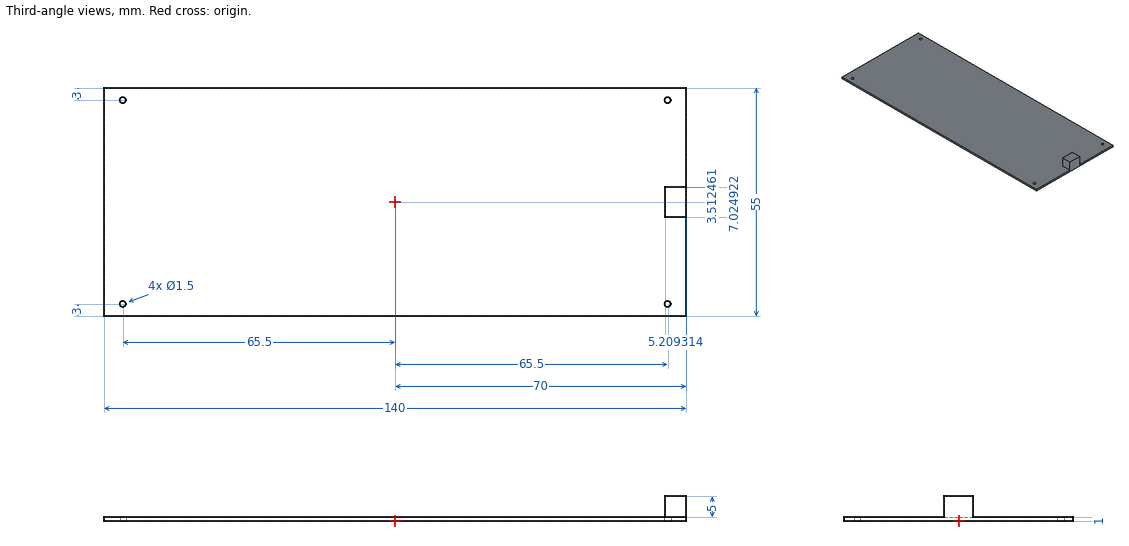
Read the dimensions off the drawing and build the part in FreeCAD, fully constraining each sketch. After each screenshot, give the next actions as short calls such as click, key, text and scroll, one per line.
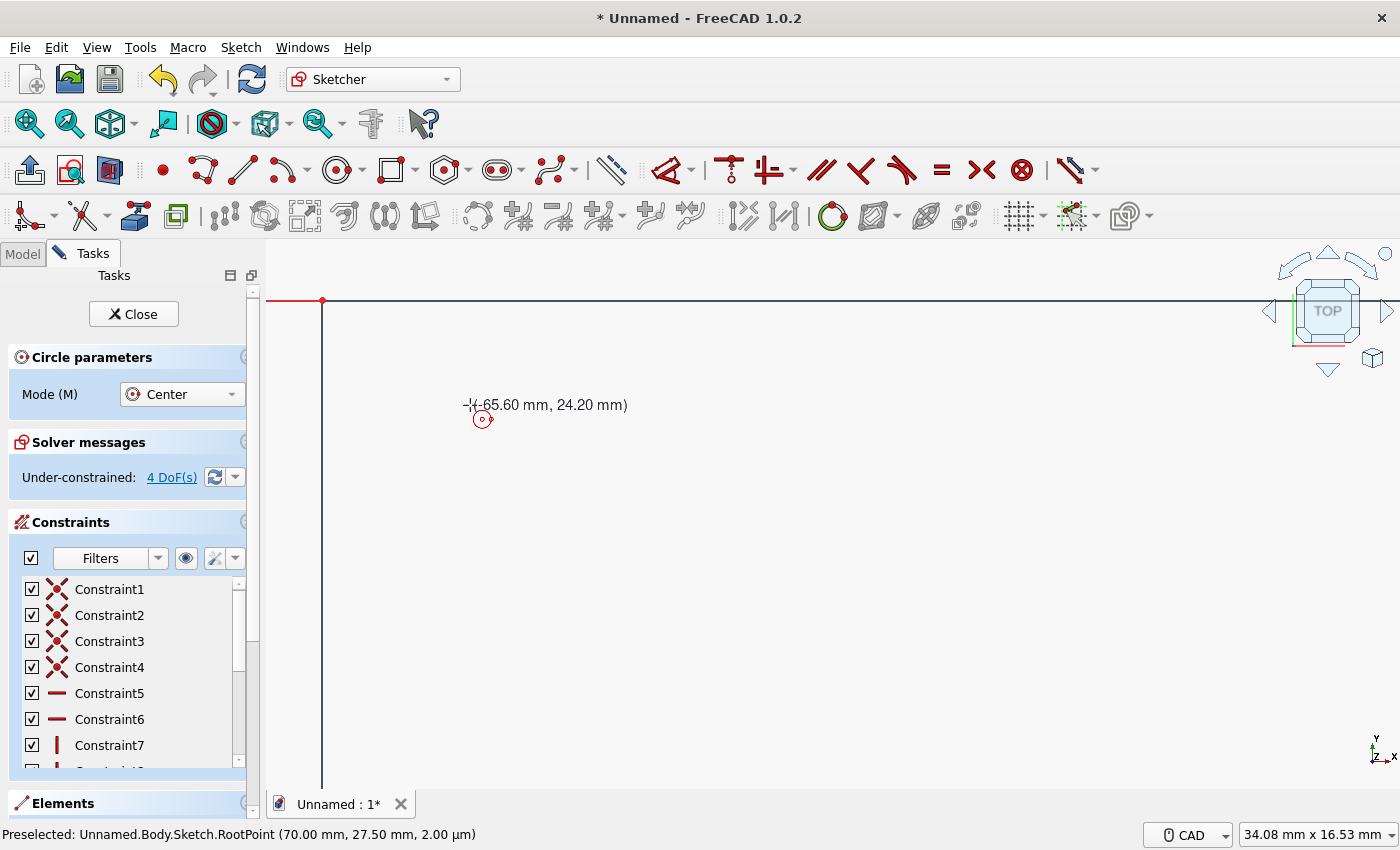
scroll(469, 404, down, 10)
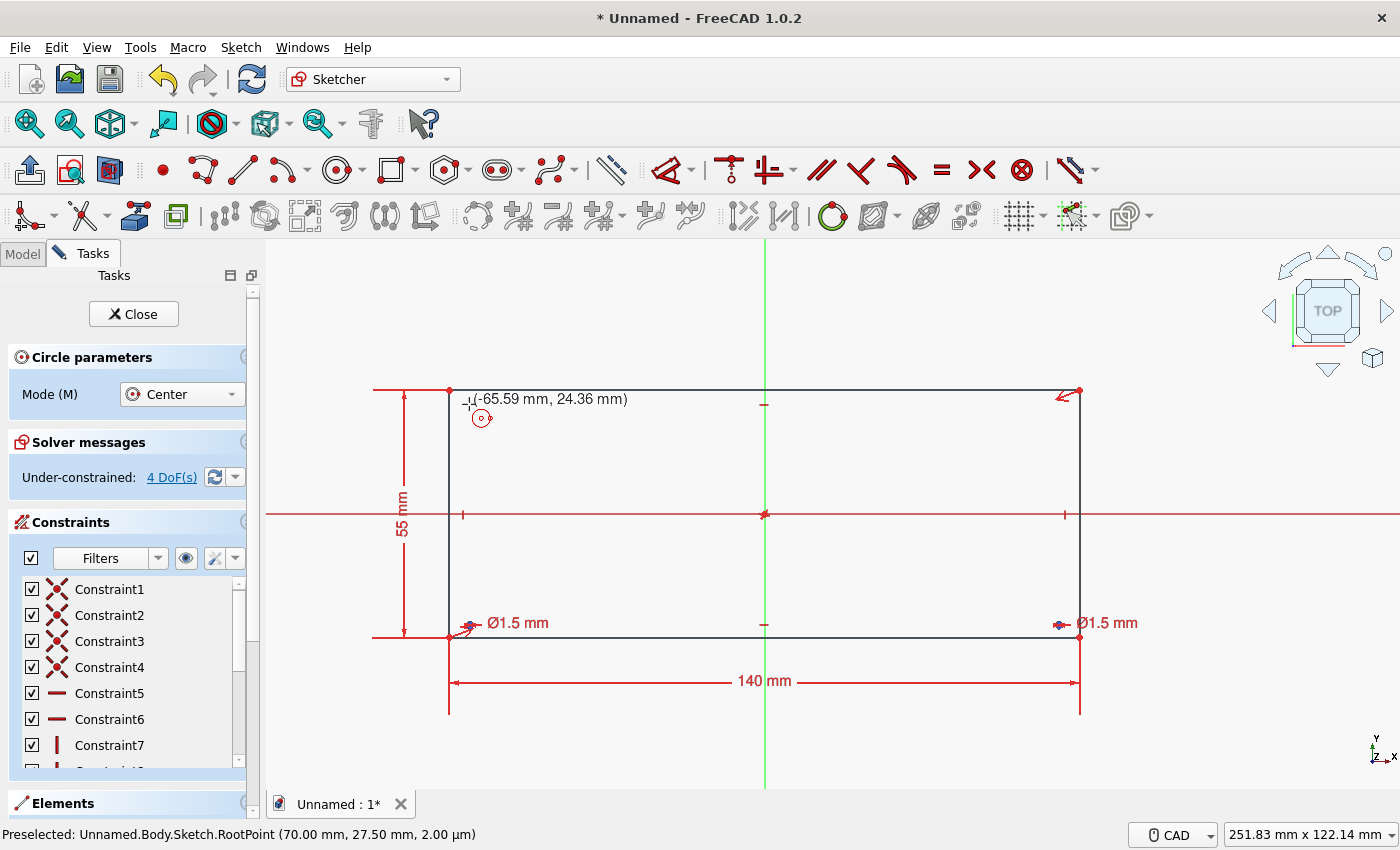
click(470, 404)
move(472, 406)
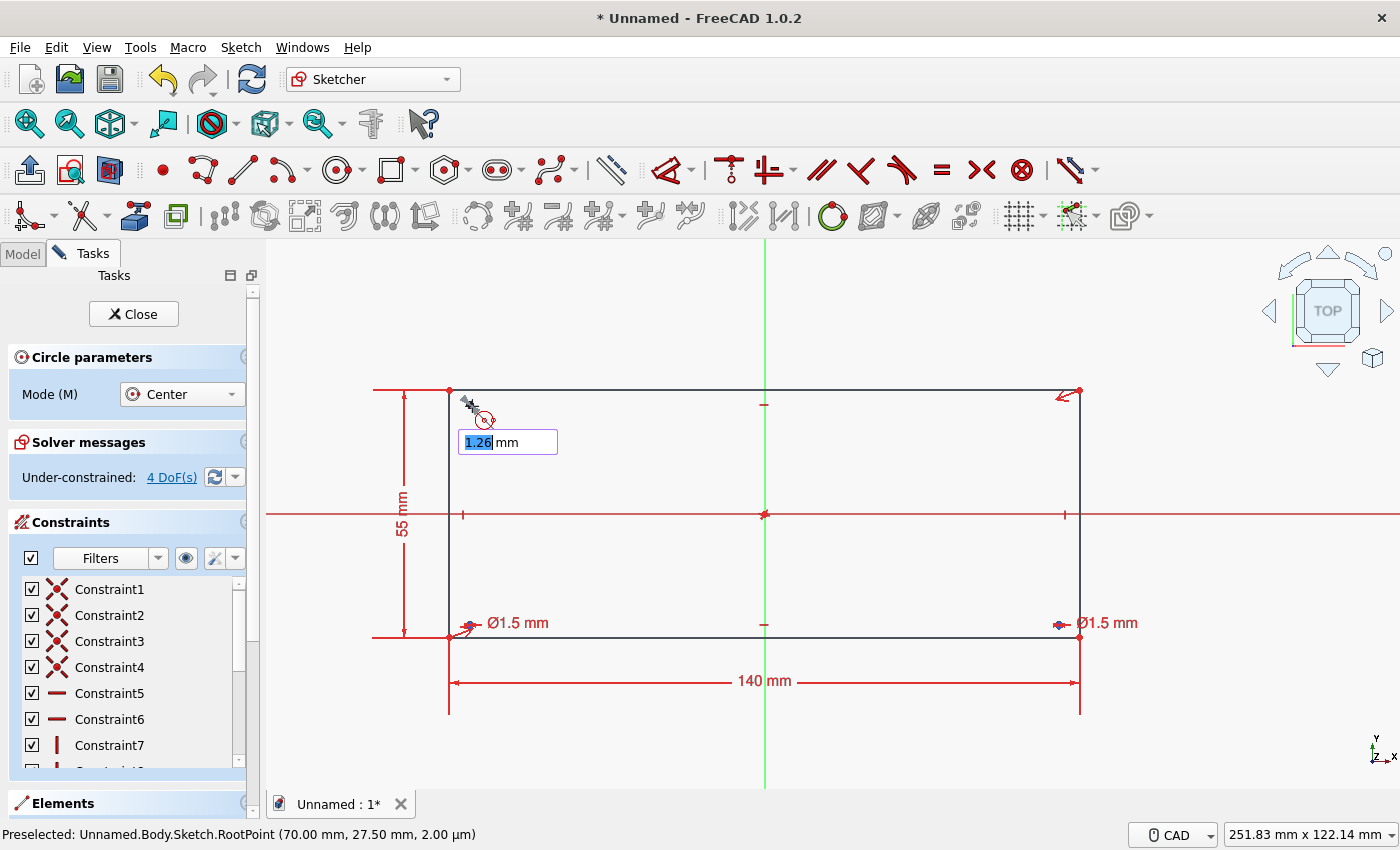
text(1.5)
key(Return)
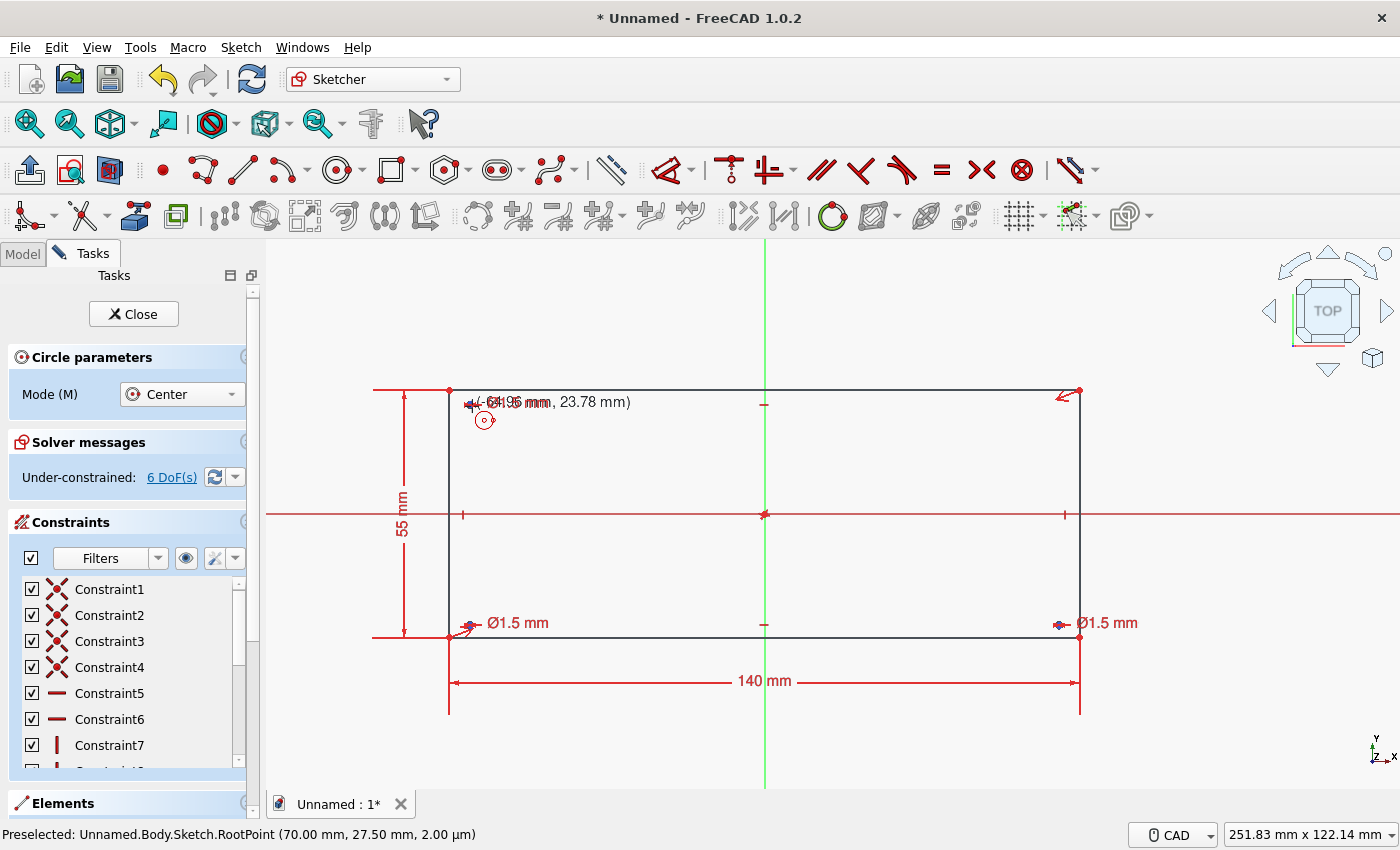
scroll(1059, 404, up, 10)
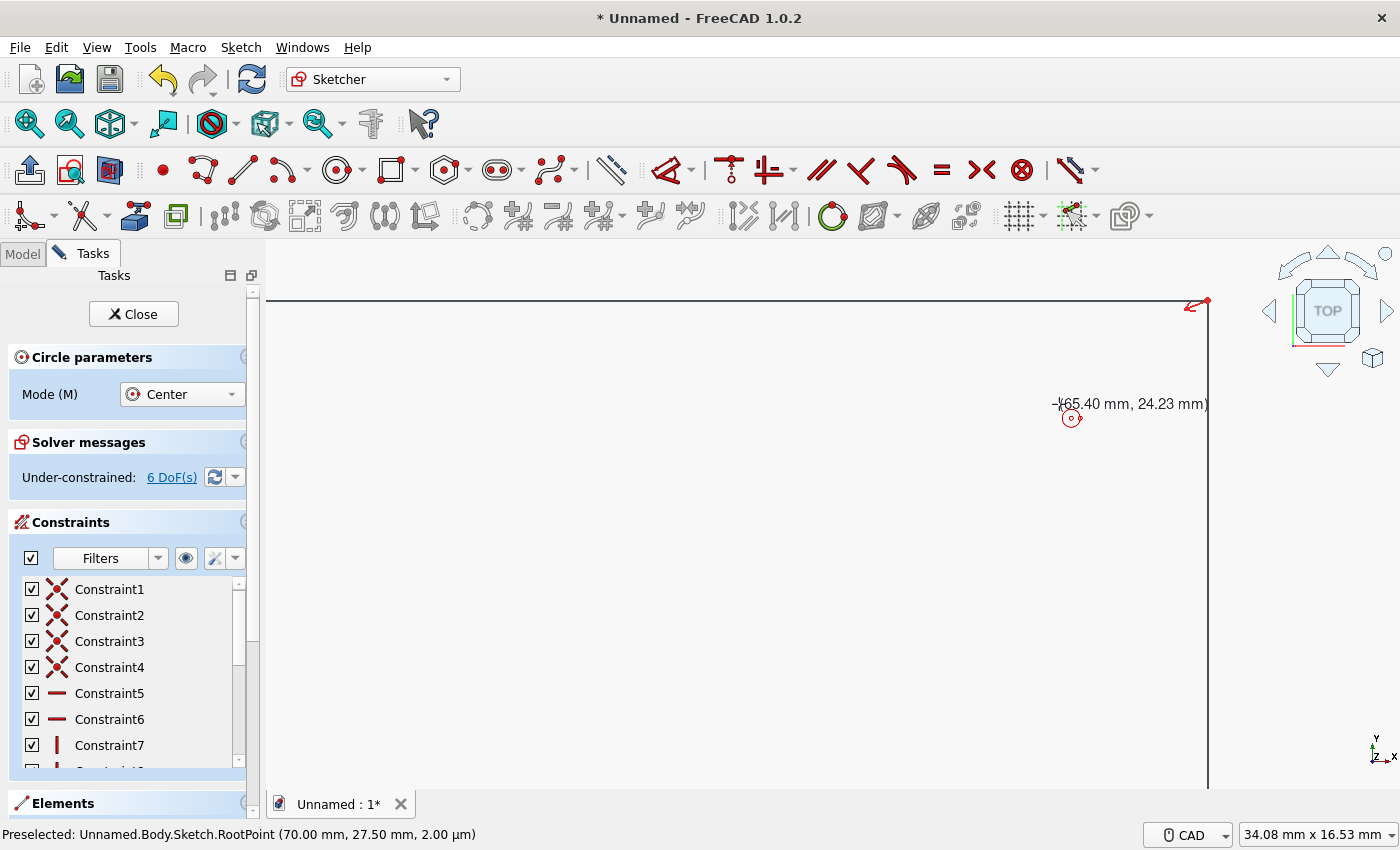
scroll(1060, 404, down, 10)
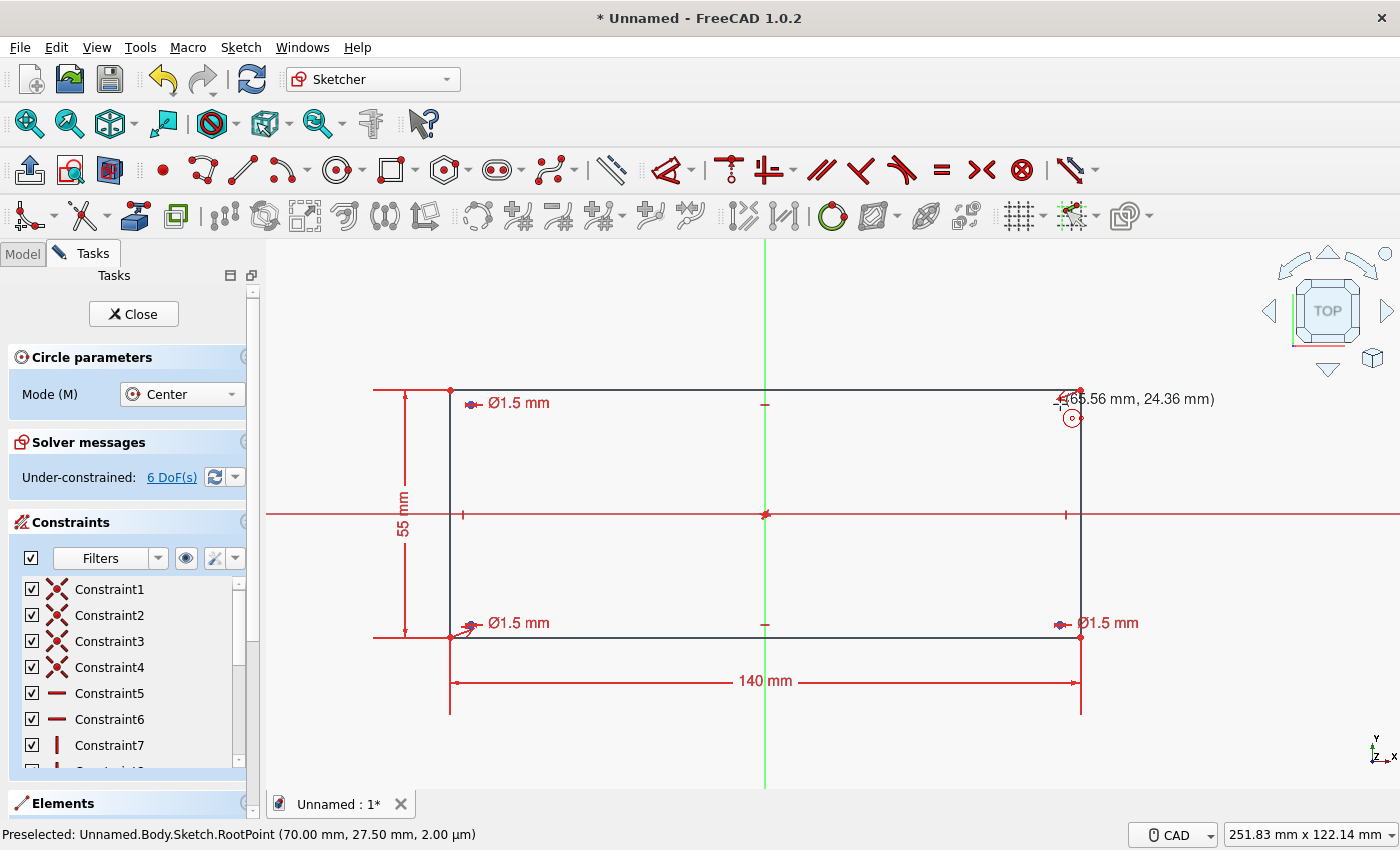
click(1060, 404)
move(1063, 406)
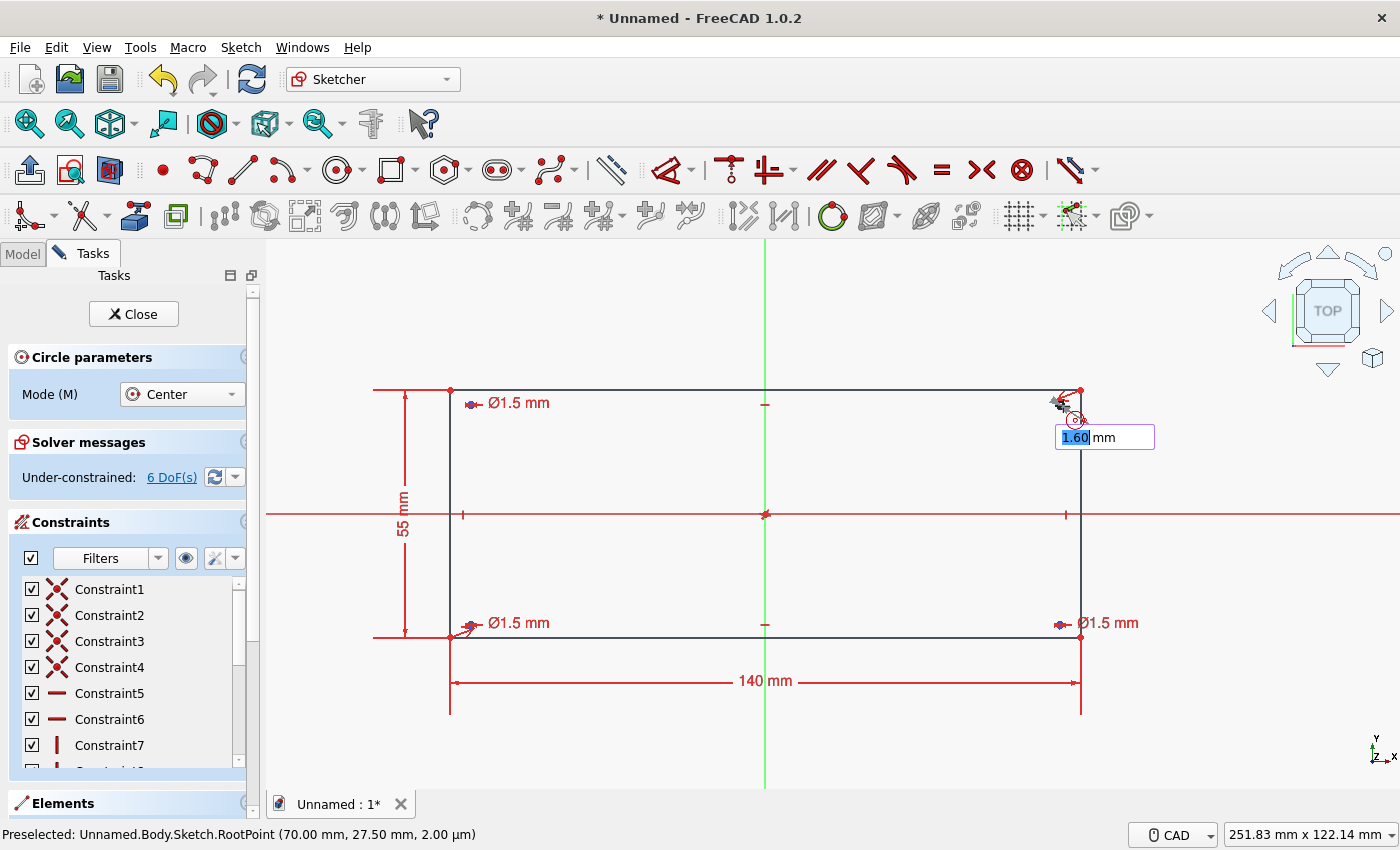
text(1.5)
key(Return)
key(Escape)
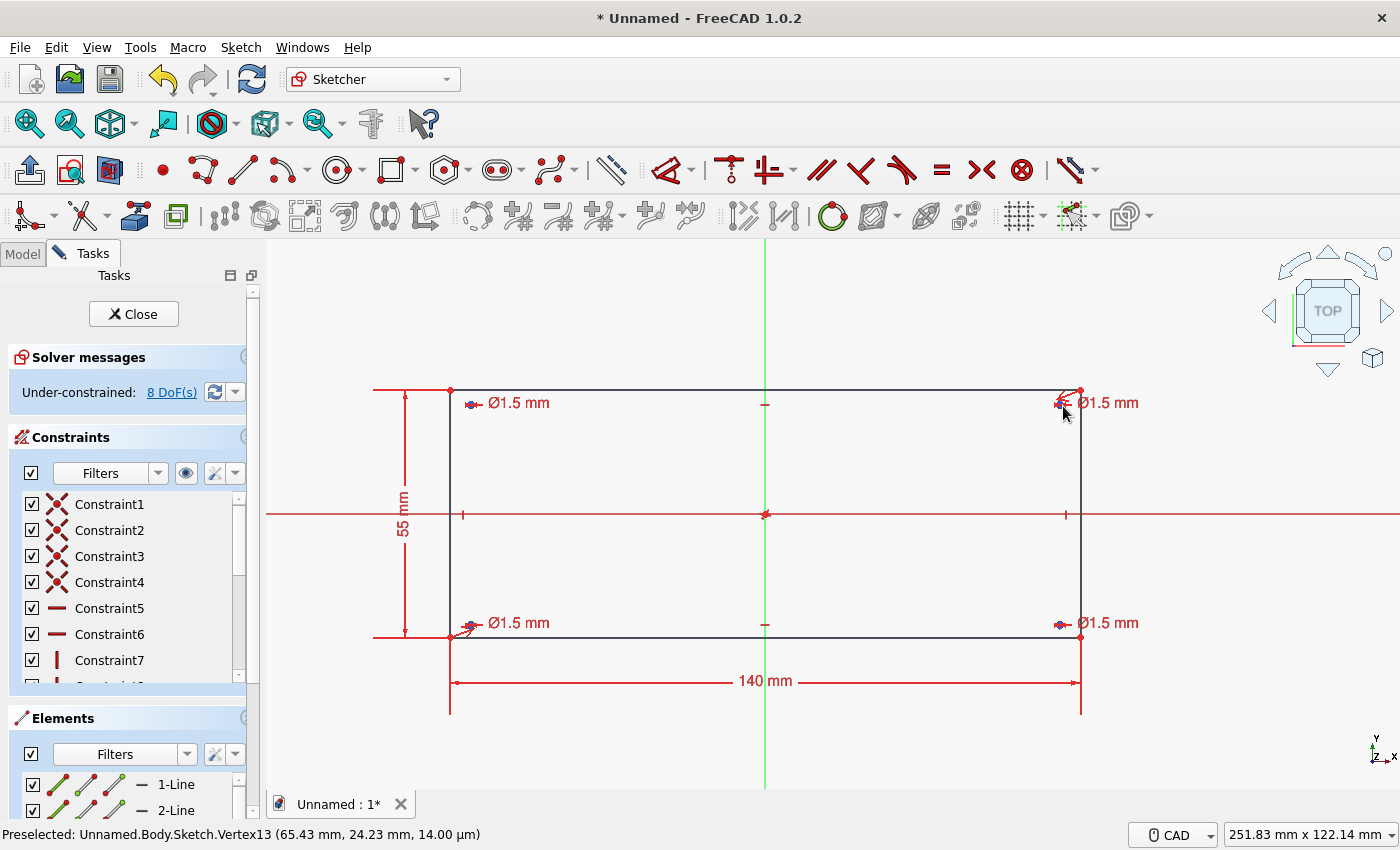
click(471, 625)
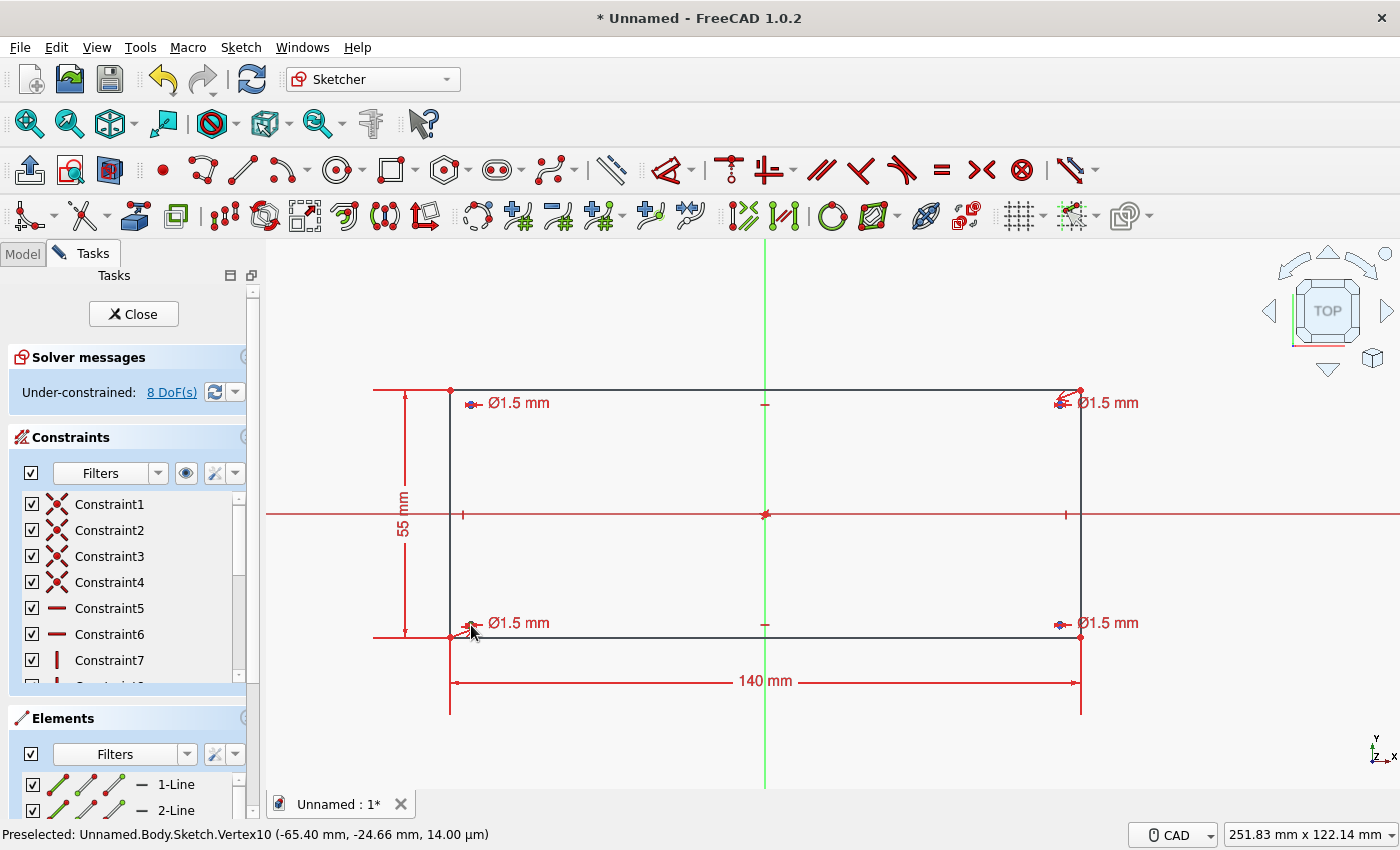
click(1060, 625)